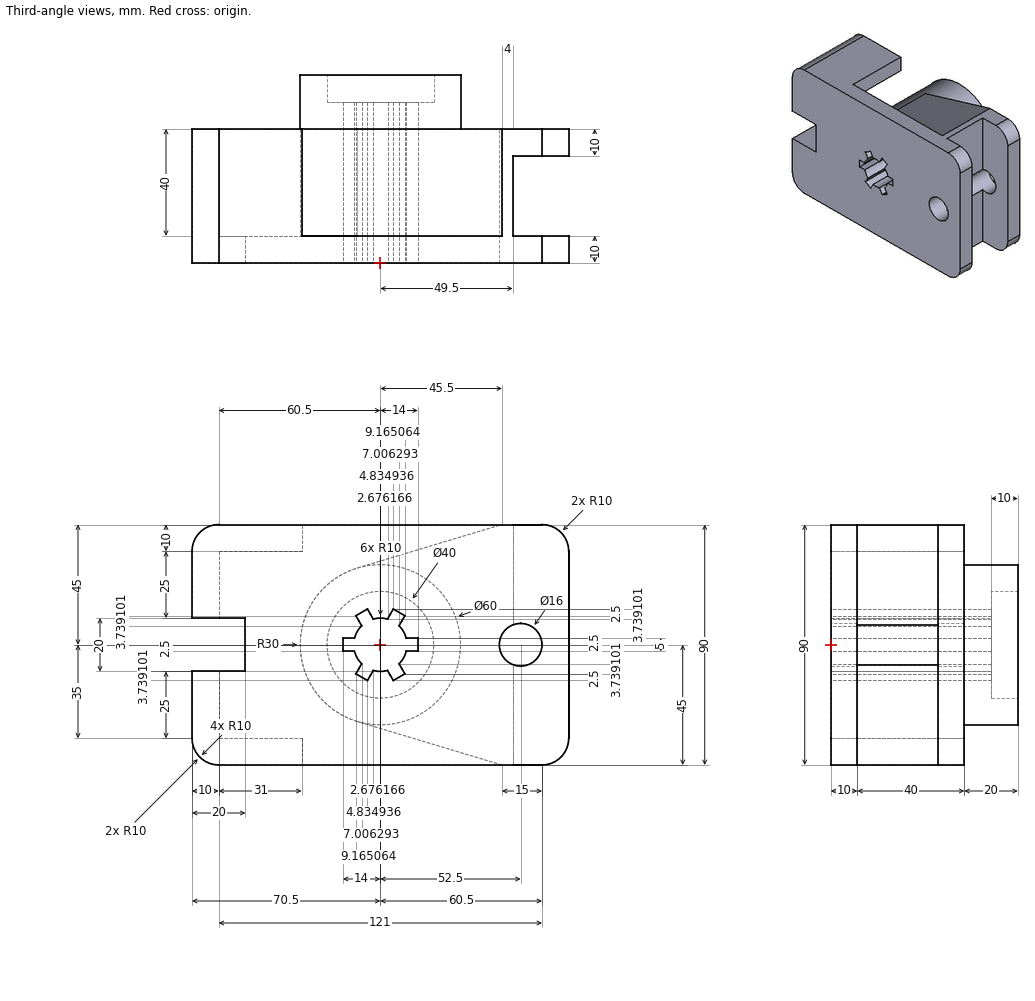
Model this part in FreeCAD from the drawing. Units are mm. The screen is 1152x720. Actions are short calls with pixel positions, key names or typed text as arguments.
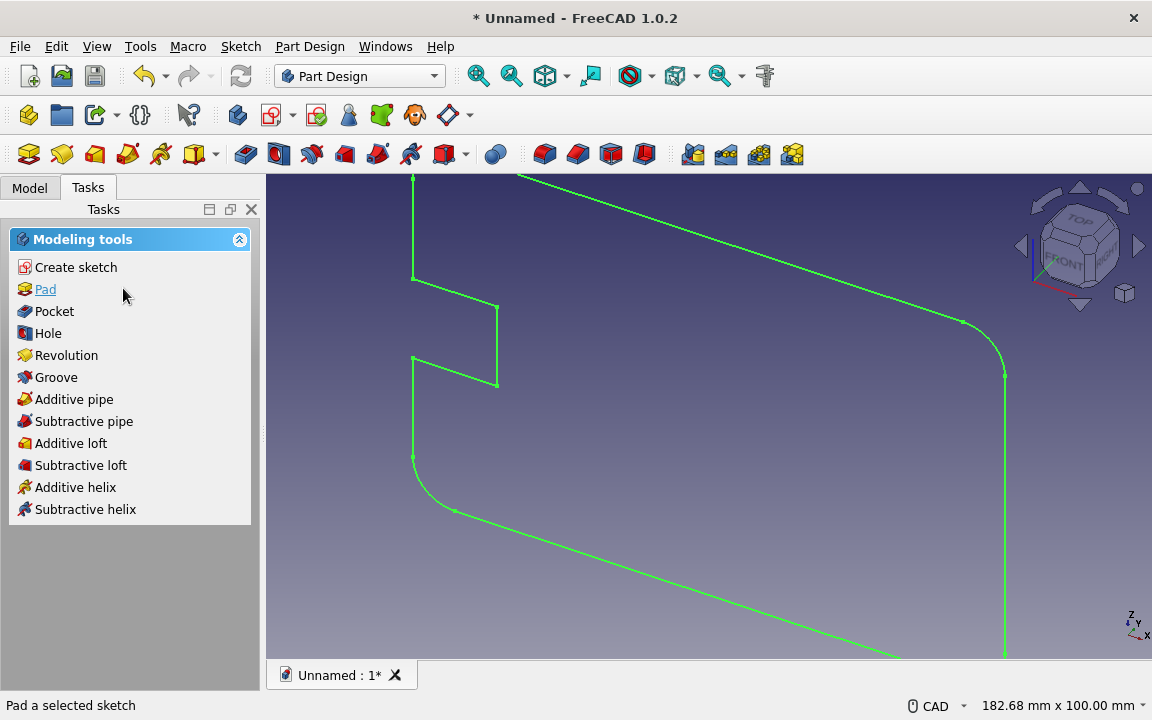
click(29, 154)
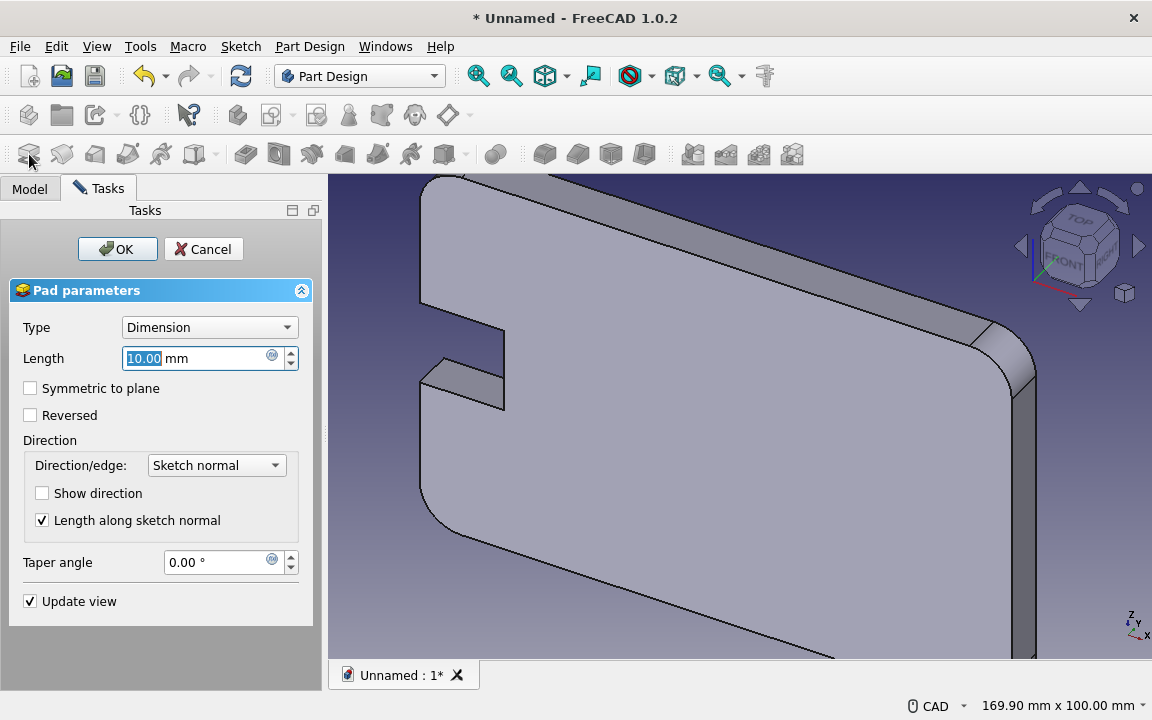
text(10)
key(Tab)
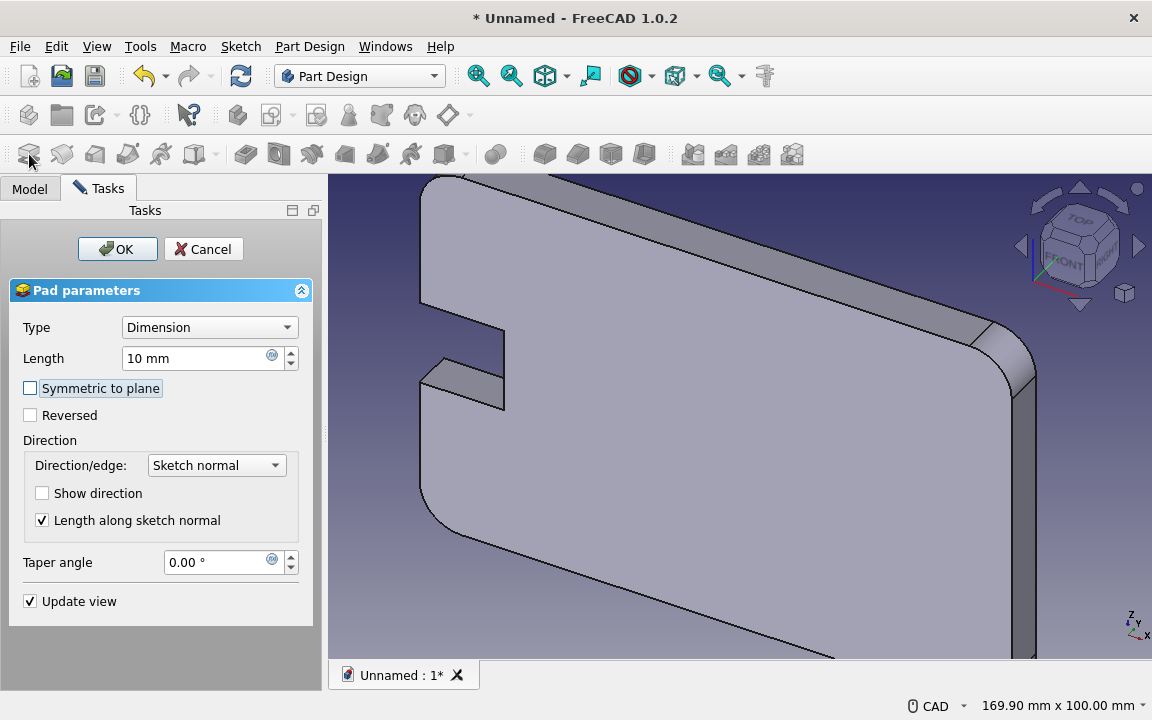
click(31, 415)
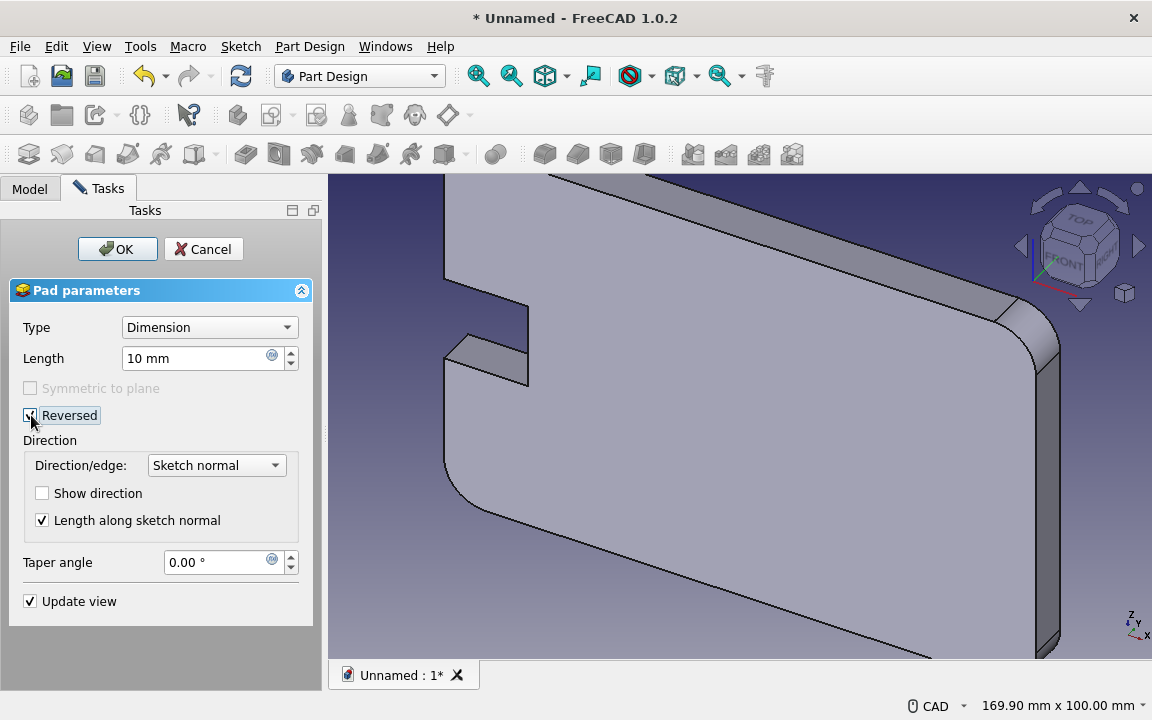
click(118, 249)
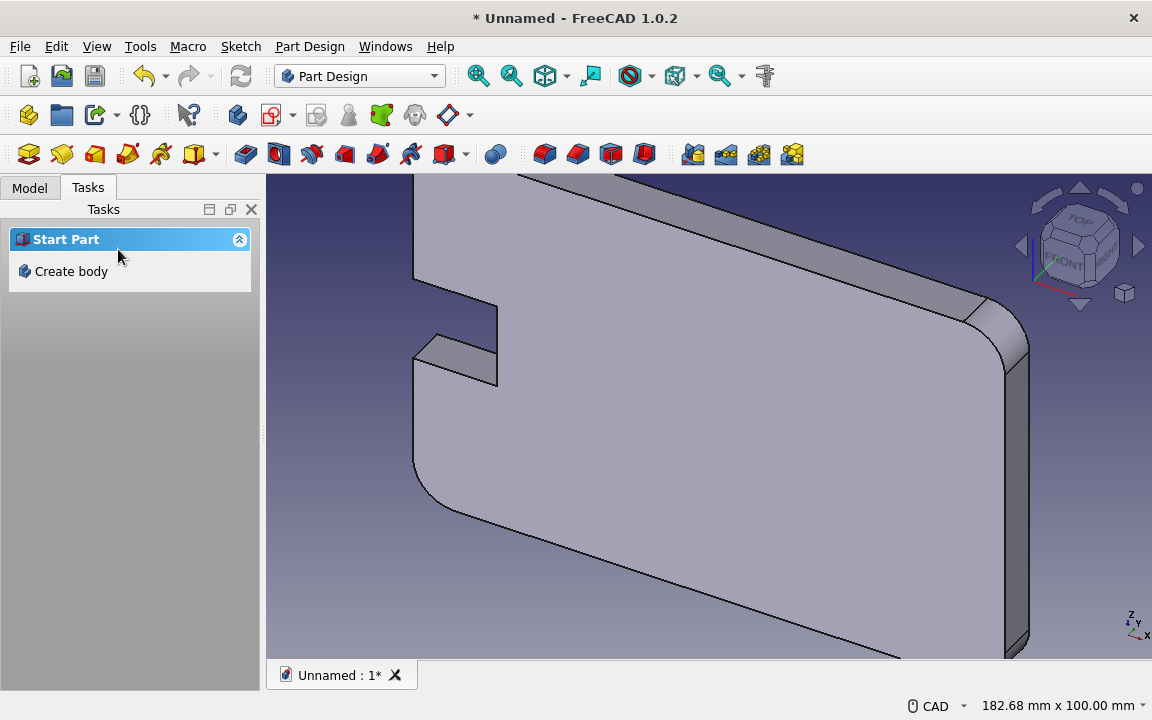
click(479, 76)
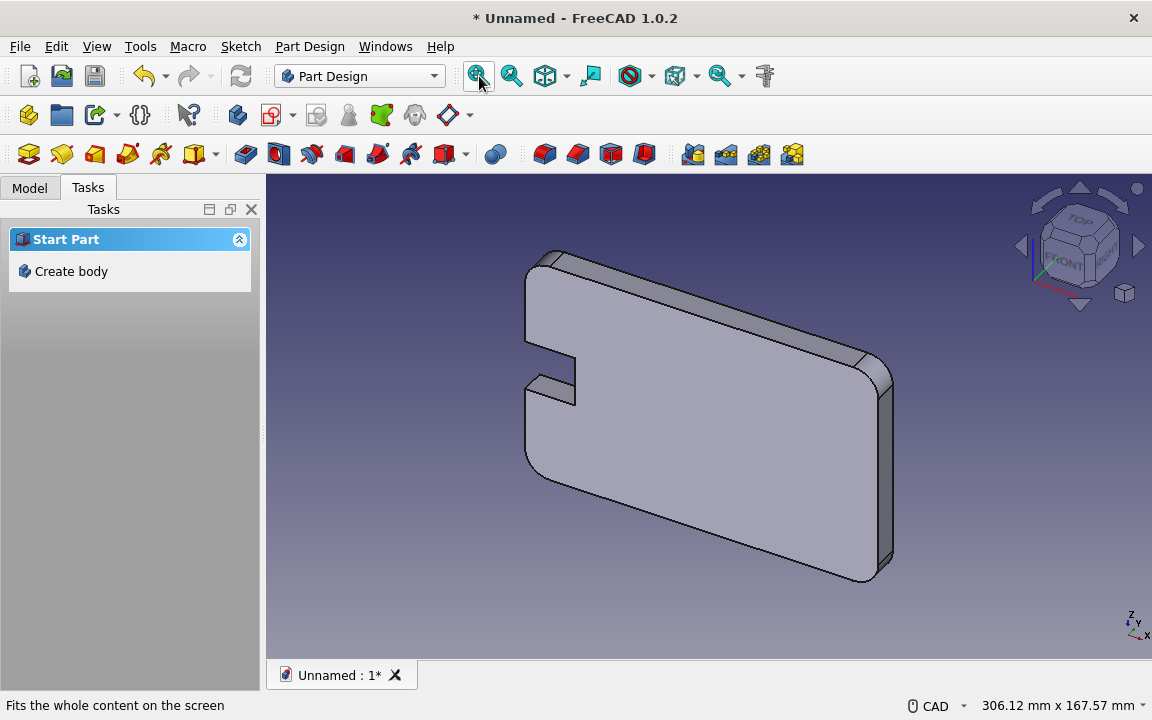
key(4)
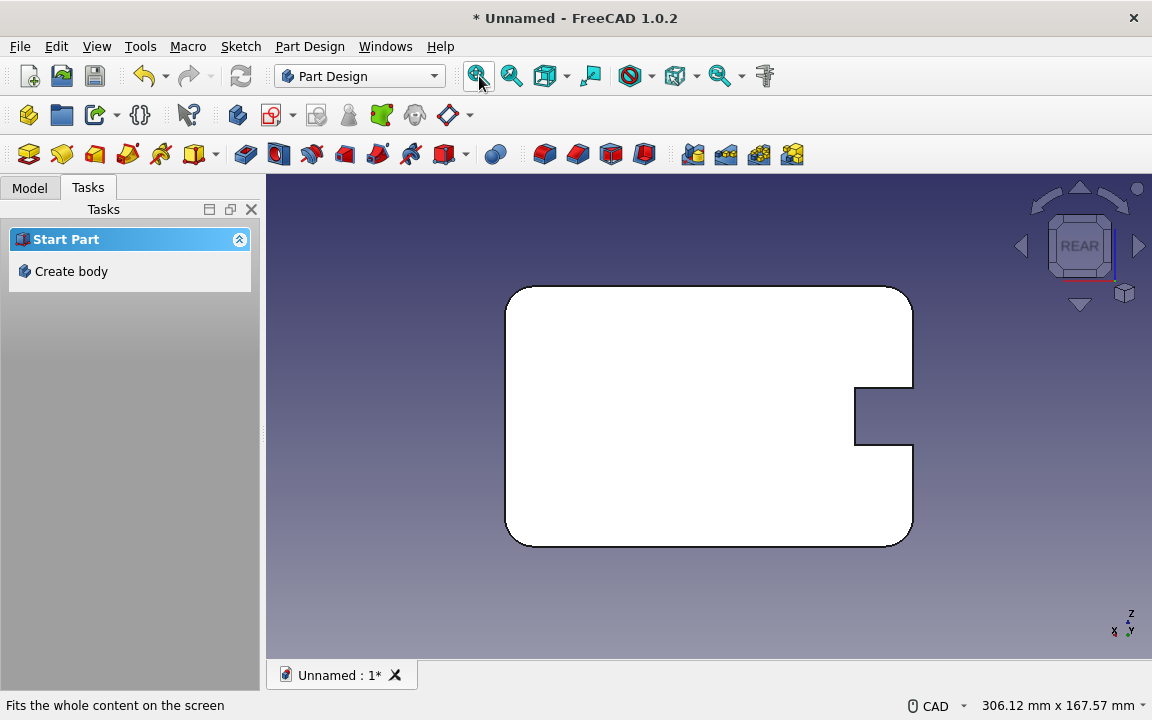
click(651, 416)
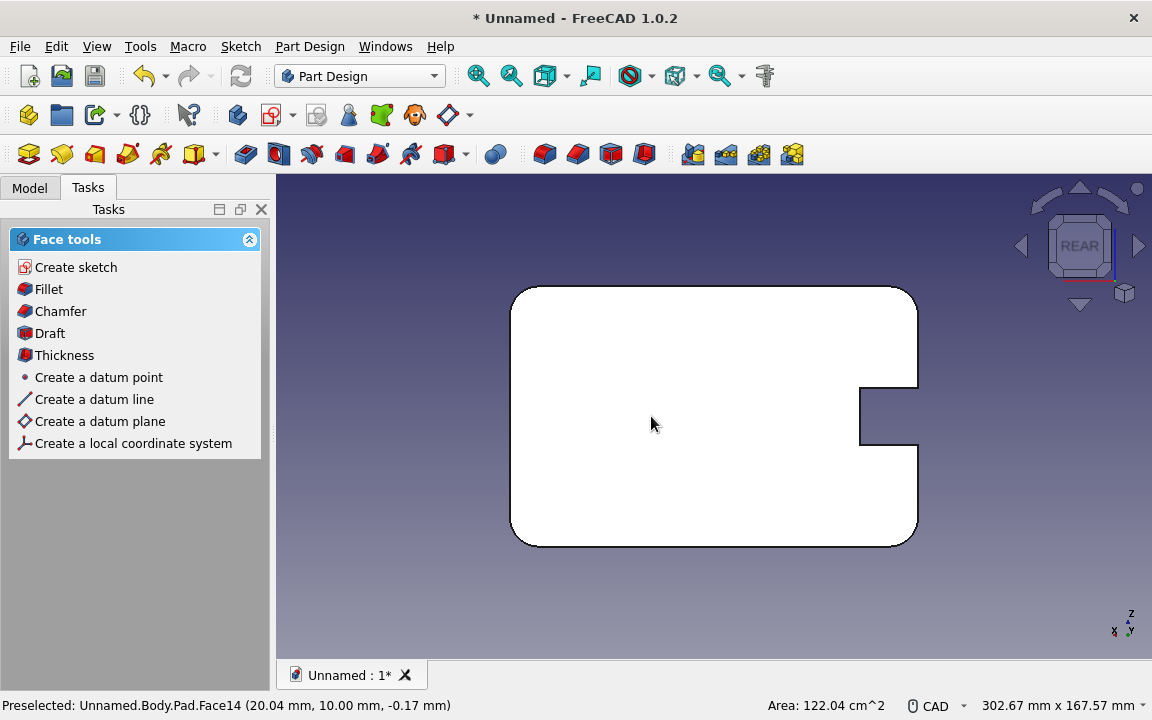
click(270, 116)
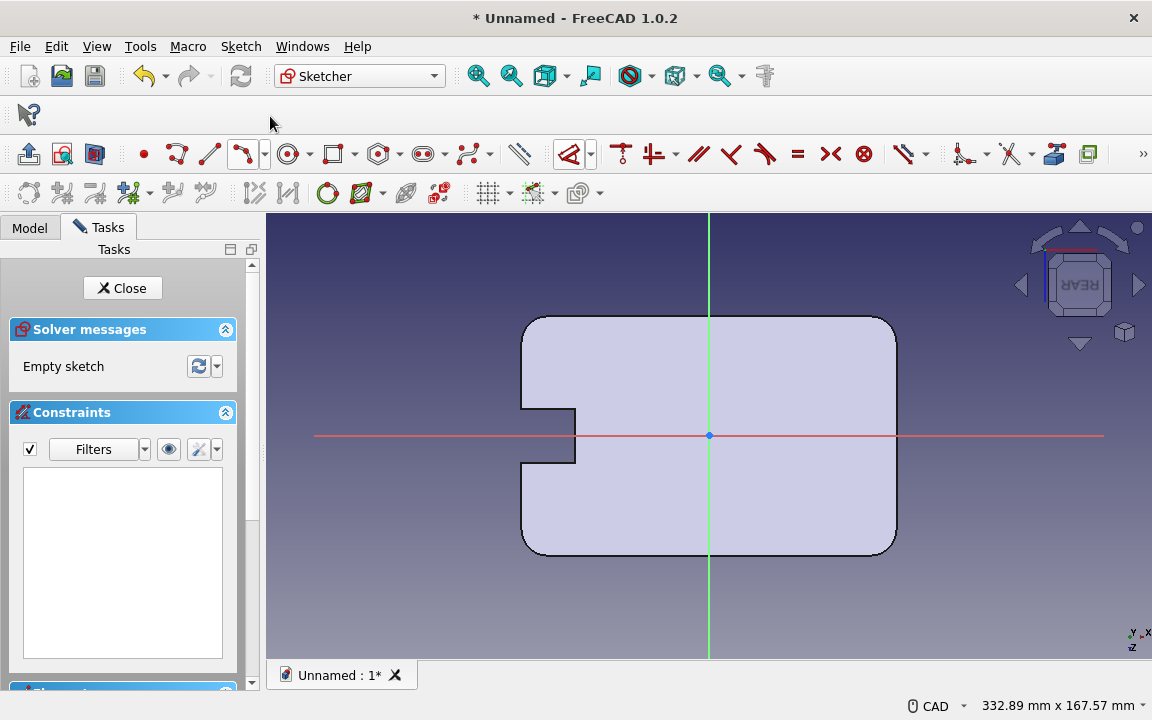
click(177, 154)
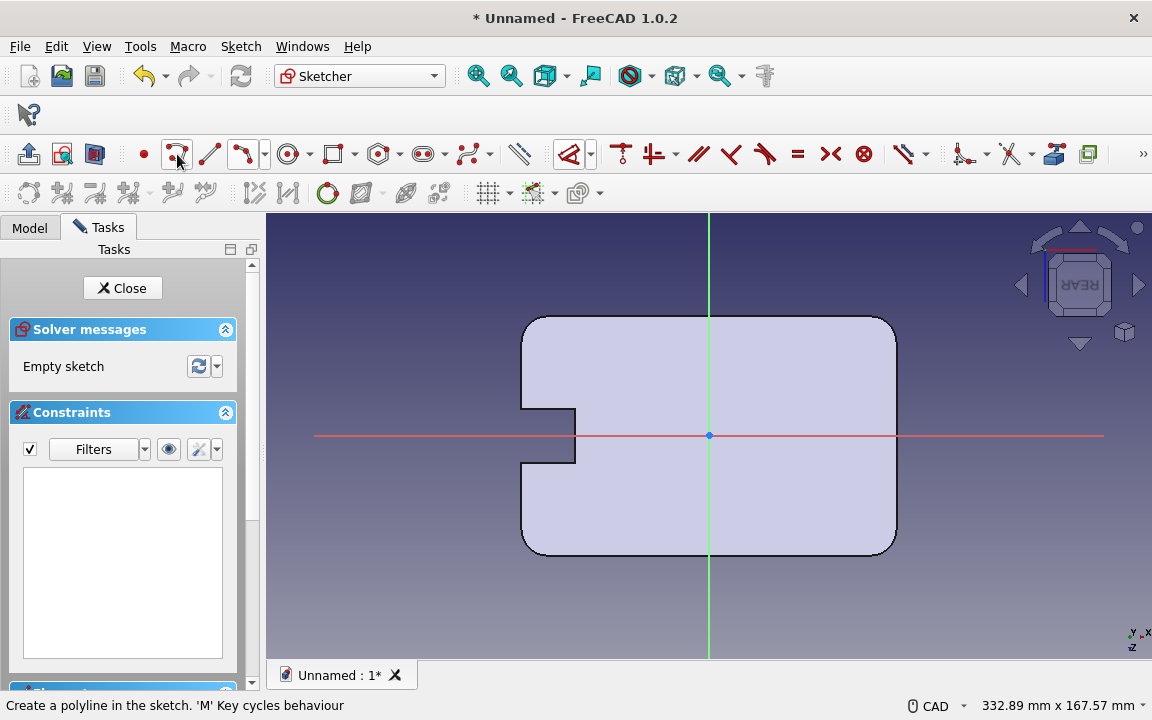
click(521, 343)
click(521, 409)
click(548, 409)
click(548, 343)
click(630, 343)
click(630, 316)
click(548, 316)
right_click(548, 316)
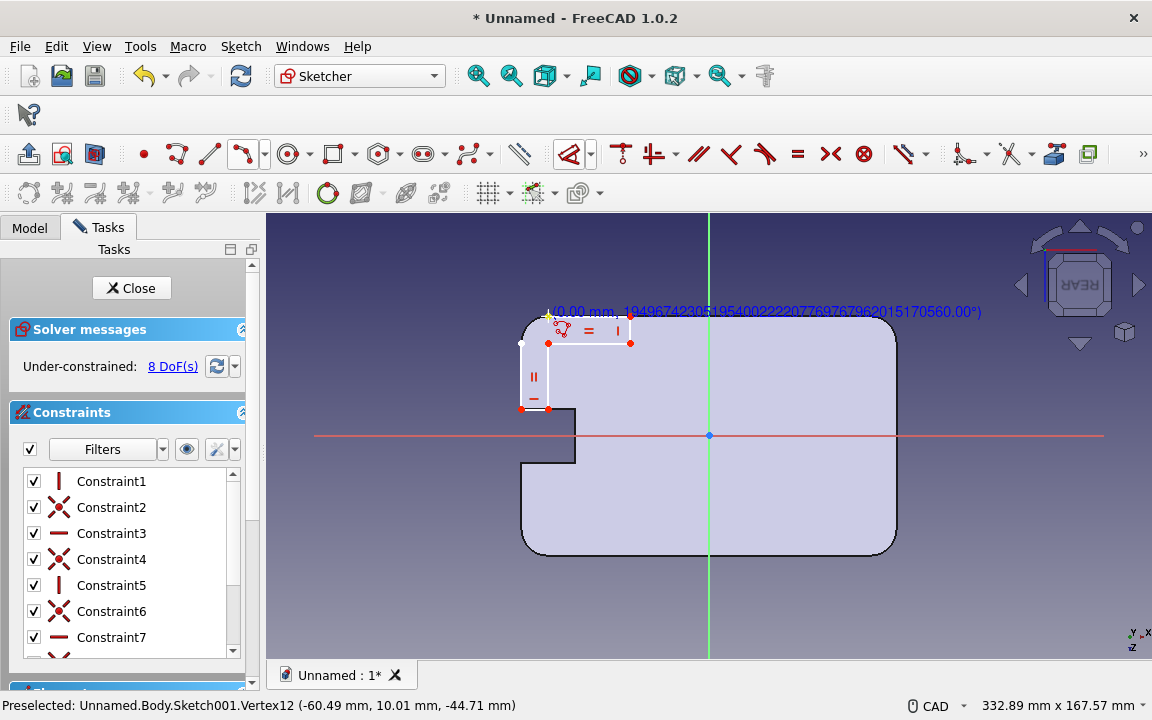
click(242, 154)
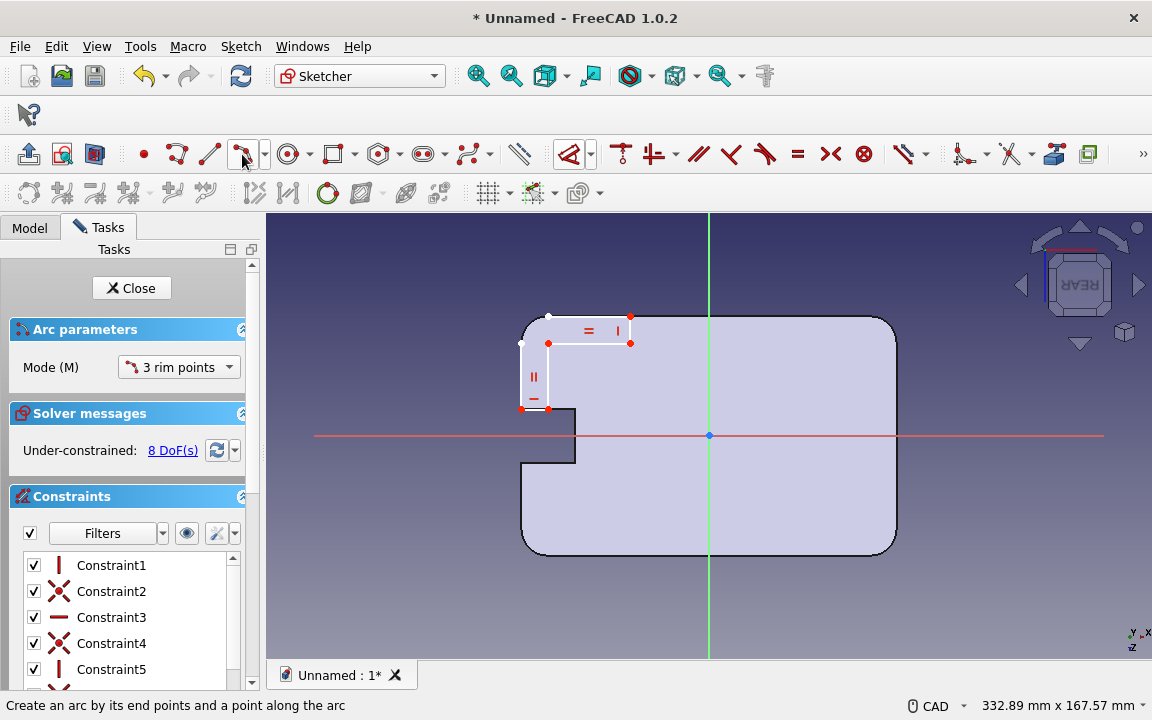
click(548, 317)
click(521, 344)